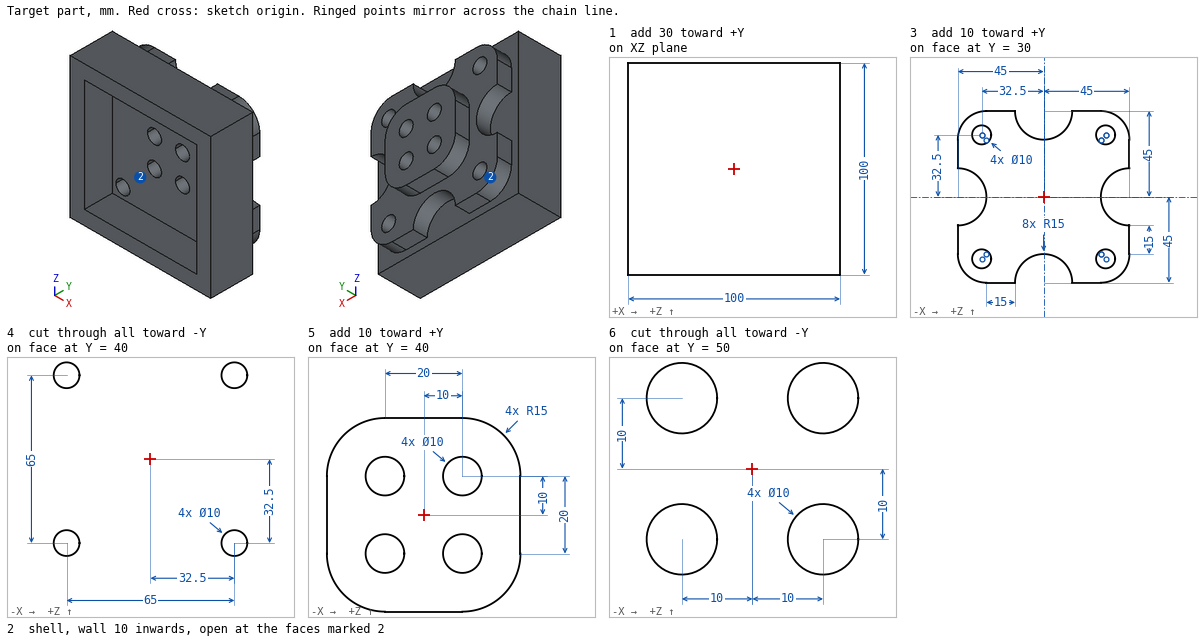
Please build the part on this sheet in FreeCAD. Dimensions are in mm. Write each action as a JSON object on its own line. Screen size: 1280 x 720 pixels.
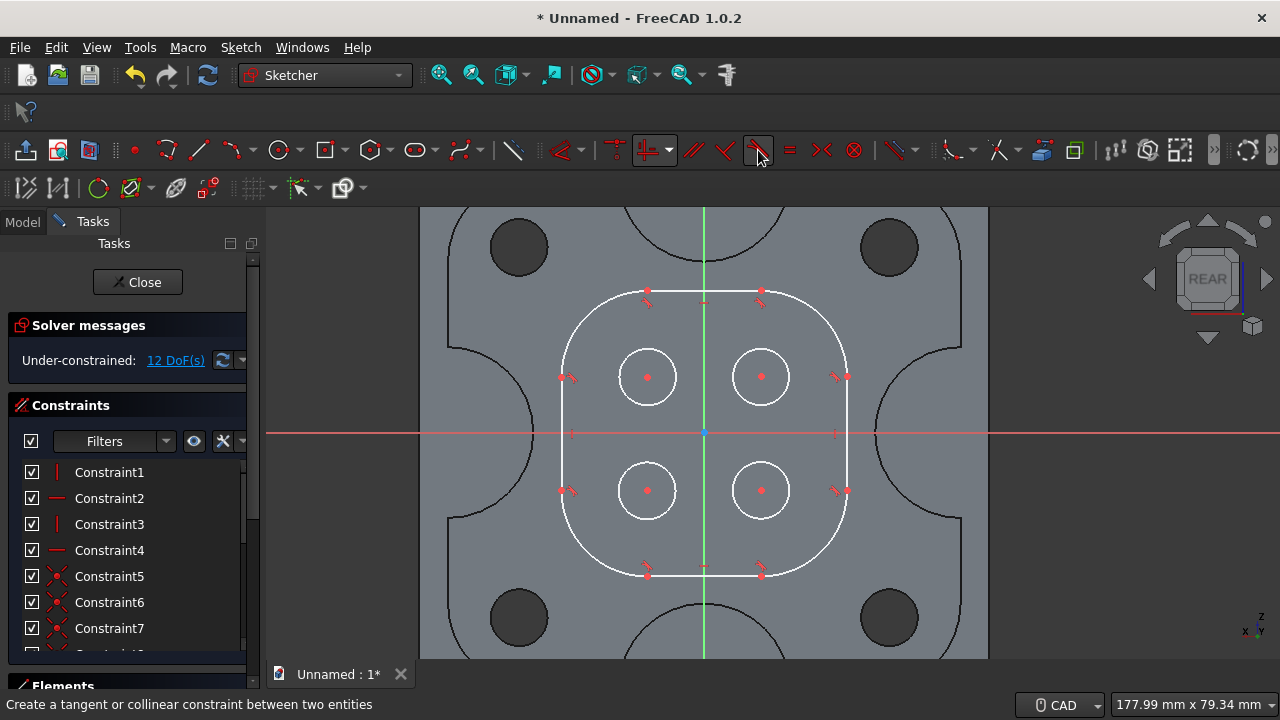
{"action": "left_click", "coordinate": [838, 338]}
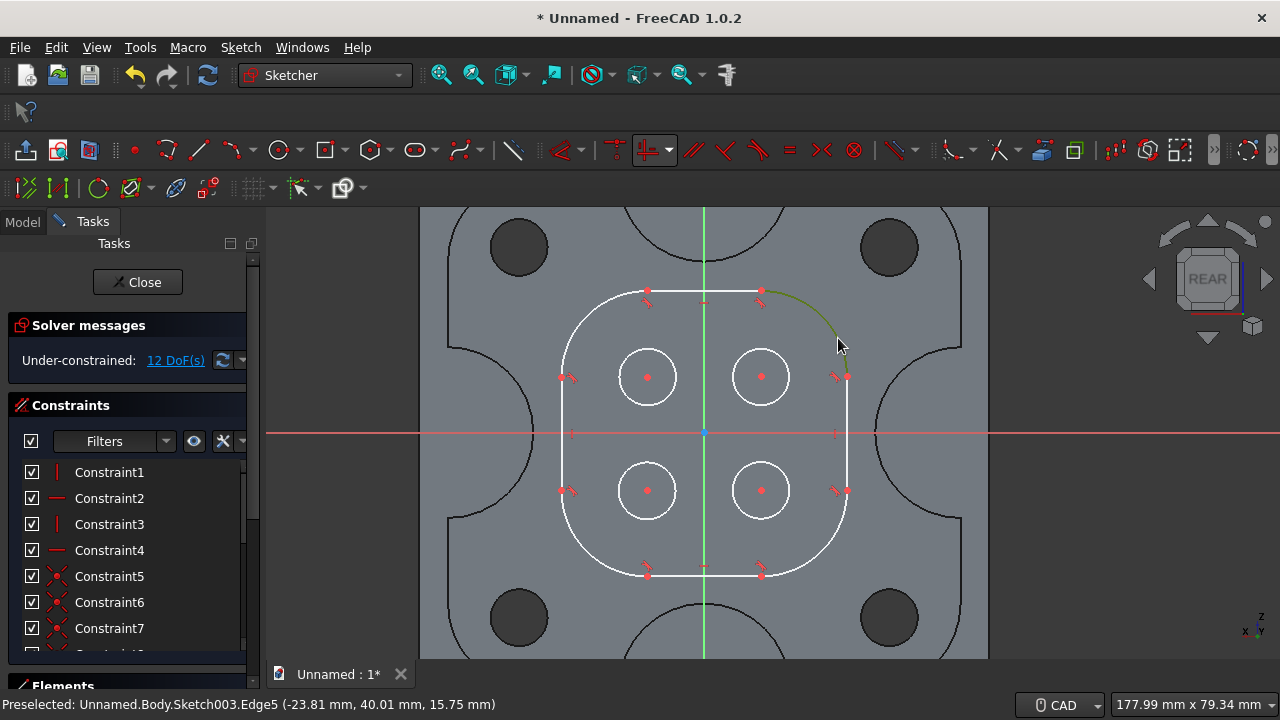
{"action": "left_click", "coordinate": [609, 300]}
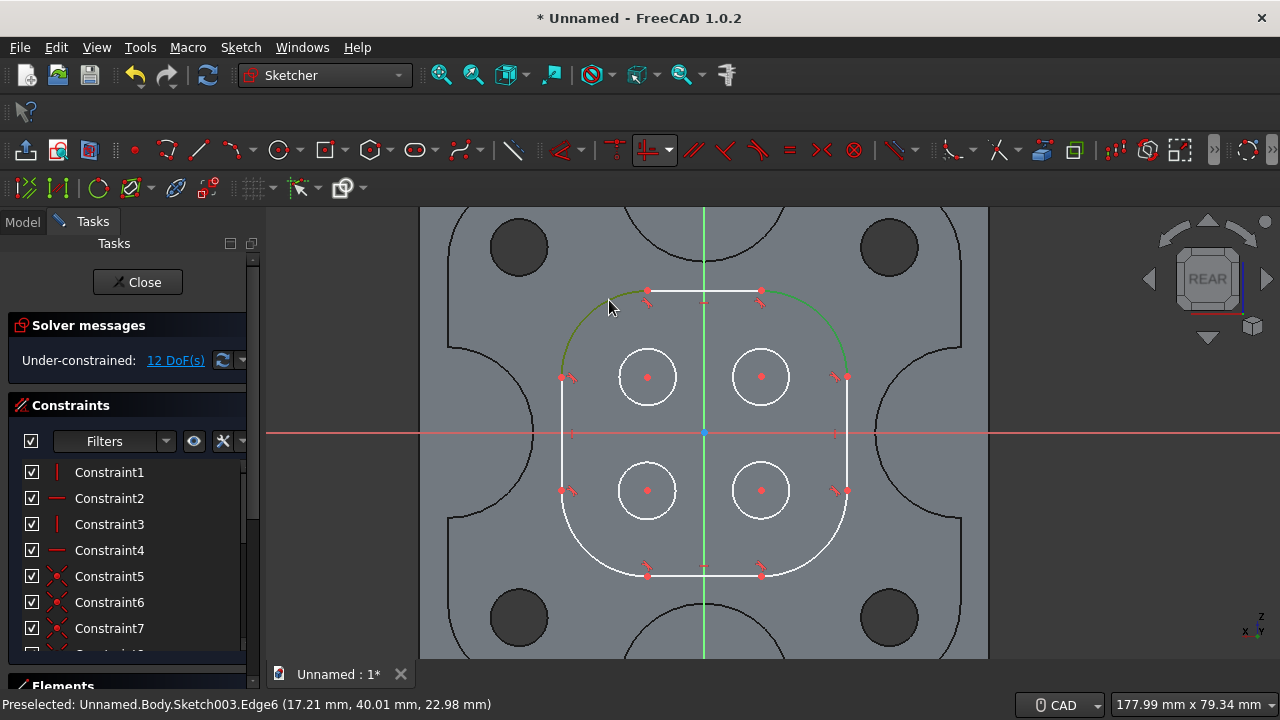
{"action": "left_click", "coordinate": [571, 530]}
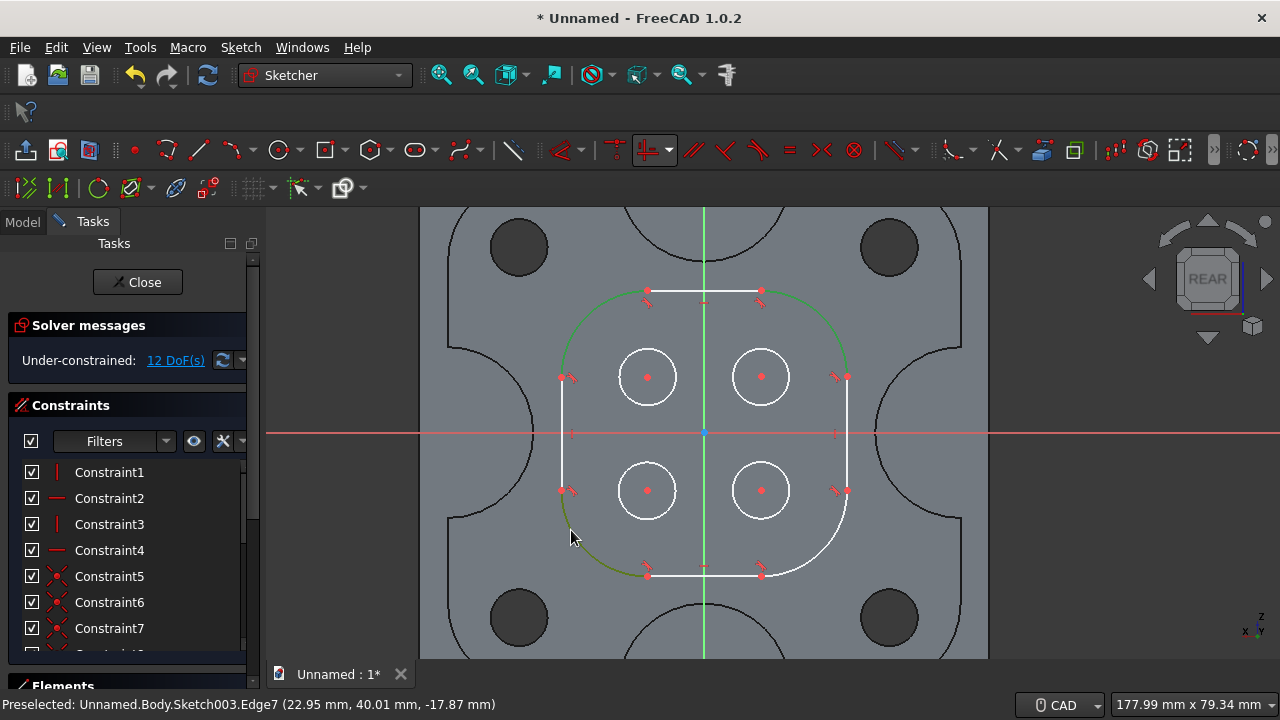
{"action": "left_click", "coordinate": [800, 567]}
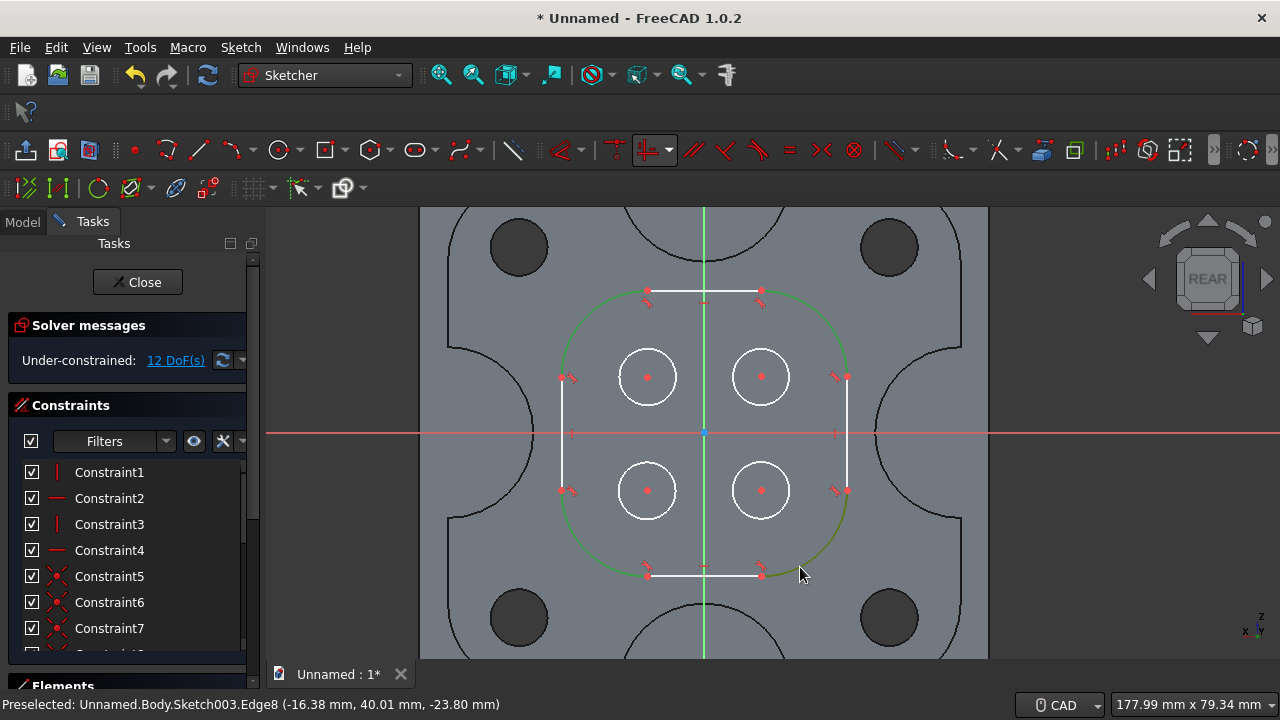
{"action": "left_click", "coordinate": [790, 150]}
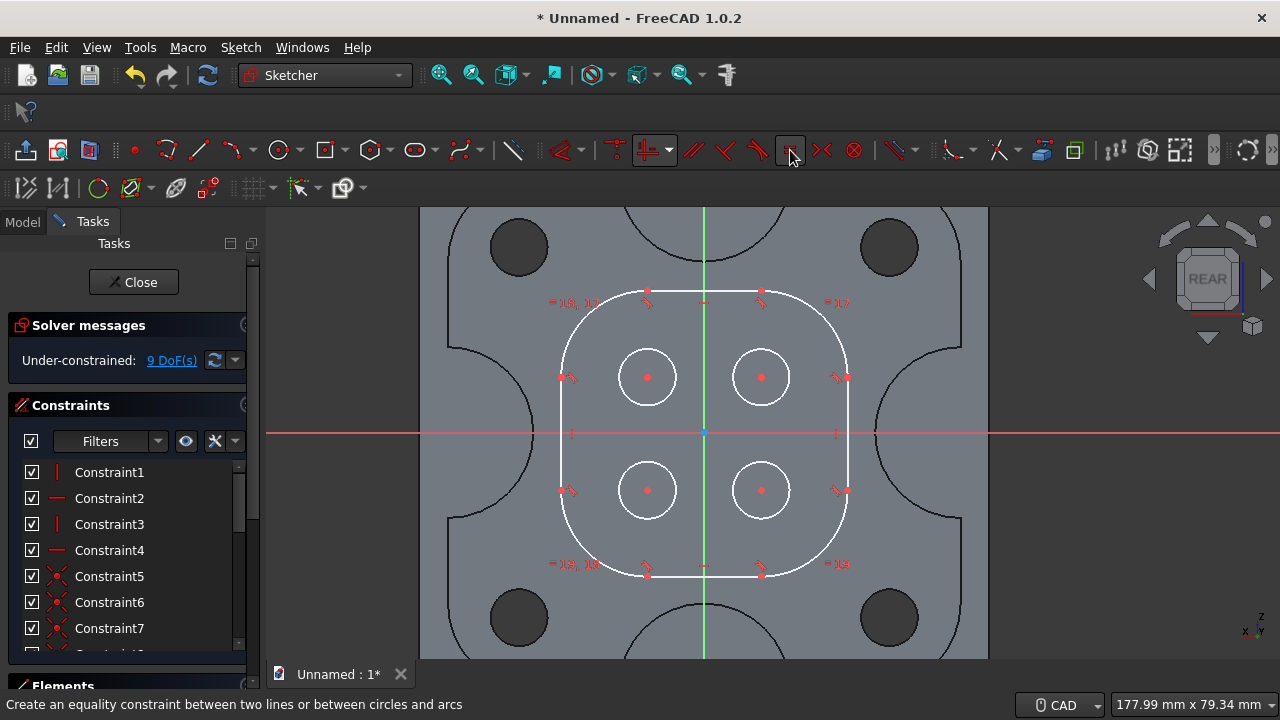
{"action": "left_click", "coordinate": [781, 357]}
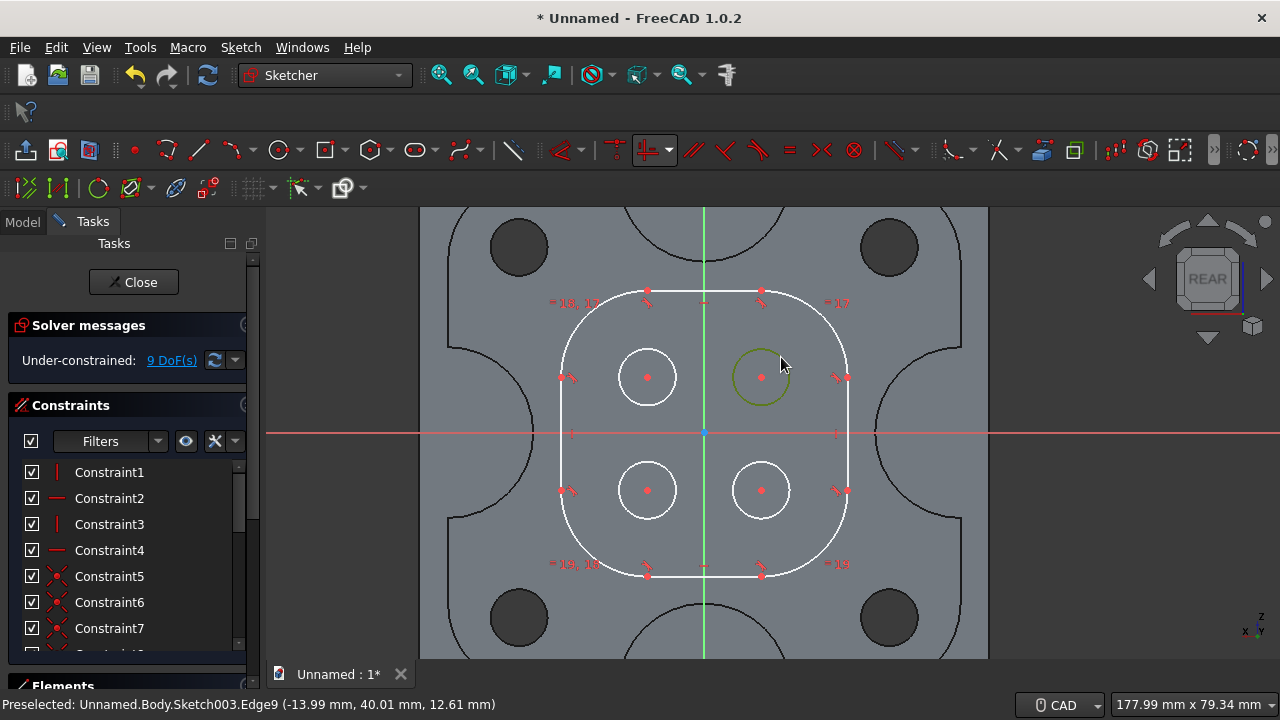
{"action": "left_click", "coordinate": [667, 357]}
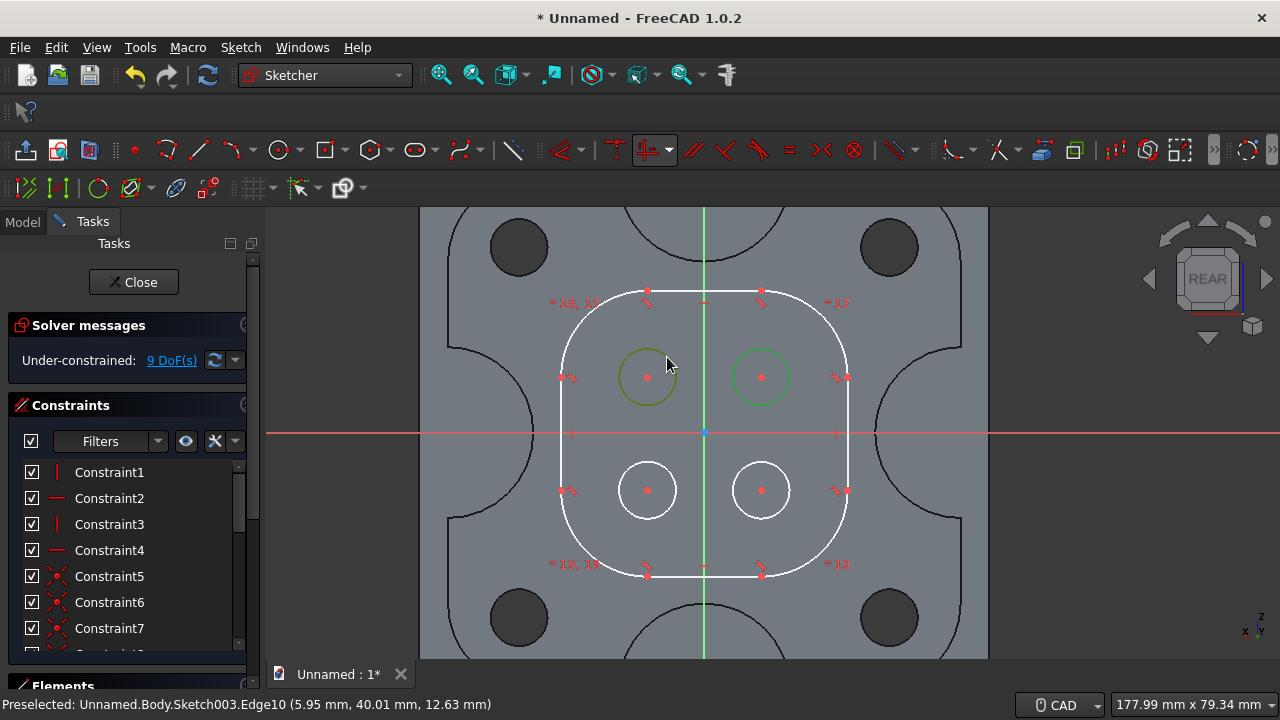
{"action": "left_click", "coordinate": [781, 470]}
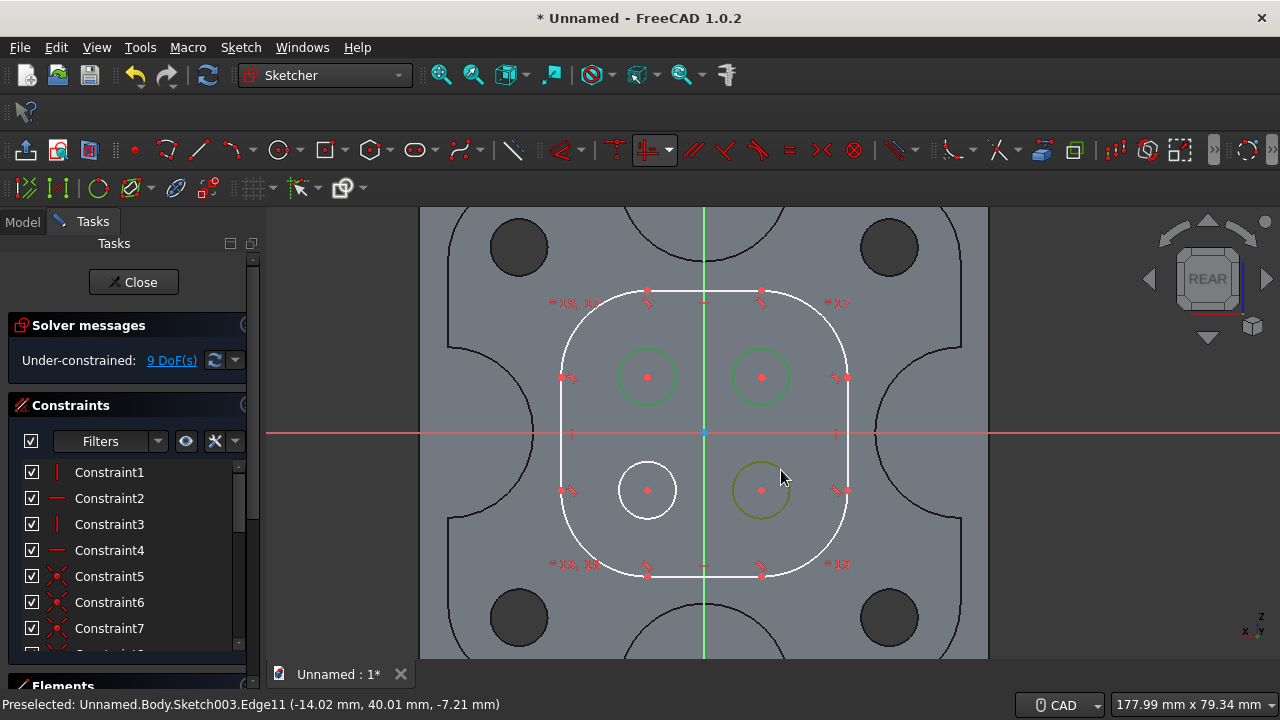
{"action": "left_click", "coordinate": [668, 470]}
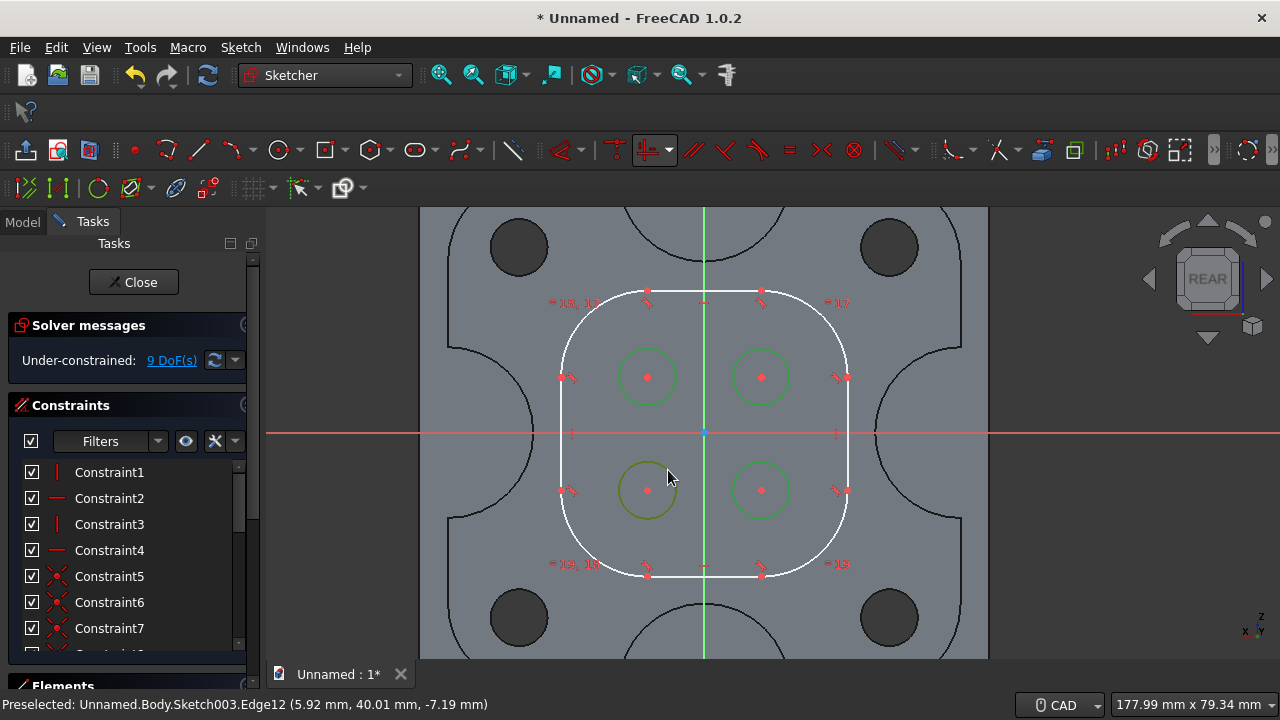
{"action": "left_click", "coordinate": [790, 150]}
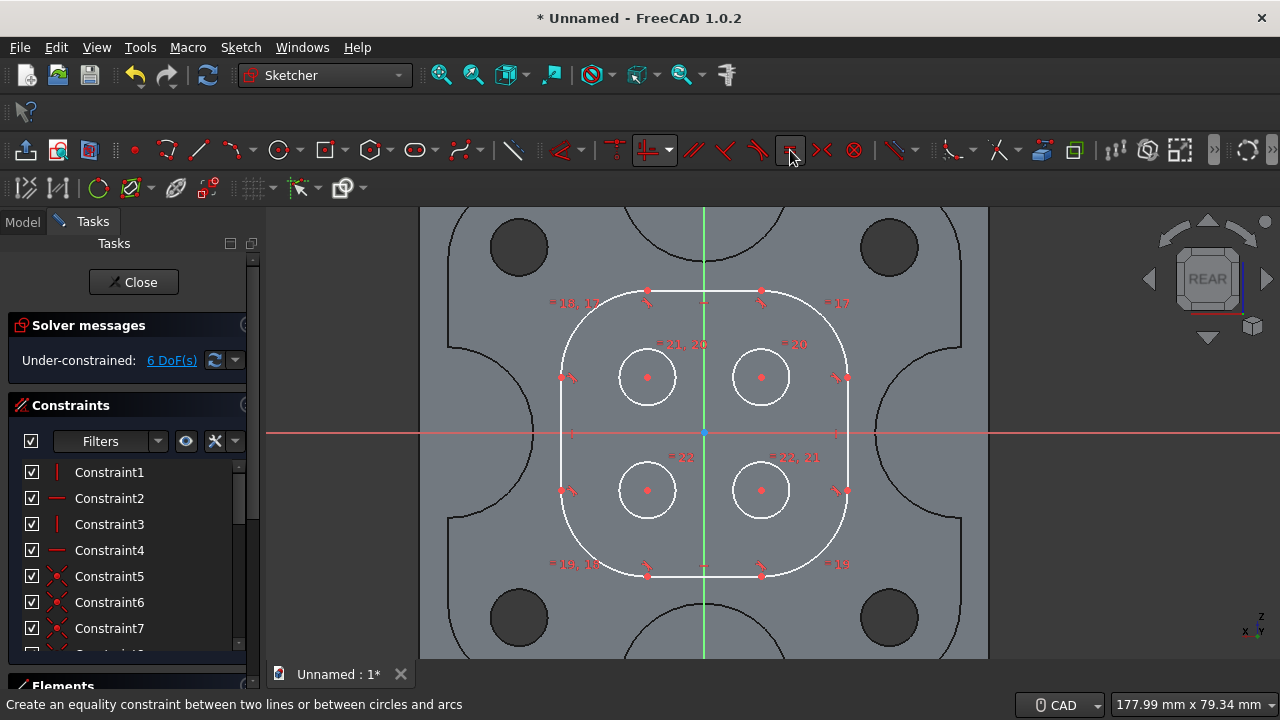
{"action": "left_click", "coordinate": [560, 150]}